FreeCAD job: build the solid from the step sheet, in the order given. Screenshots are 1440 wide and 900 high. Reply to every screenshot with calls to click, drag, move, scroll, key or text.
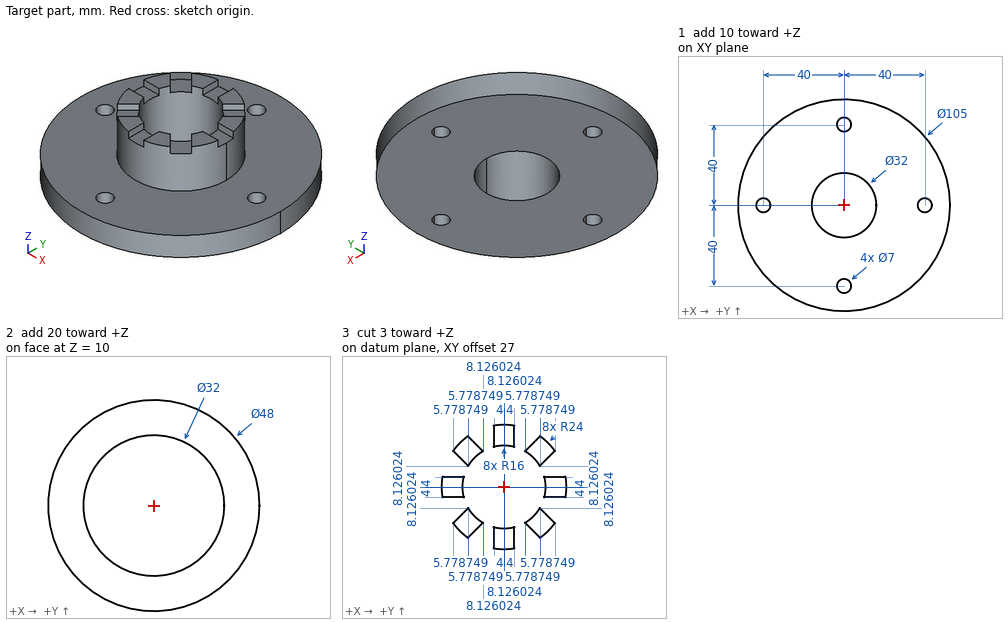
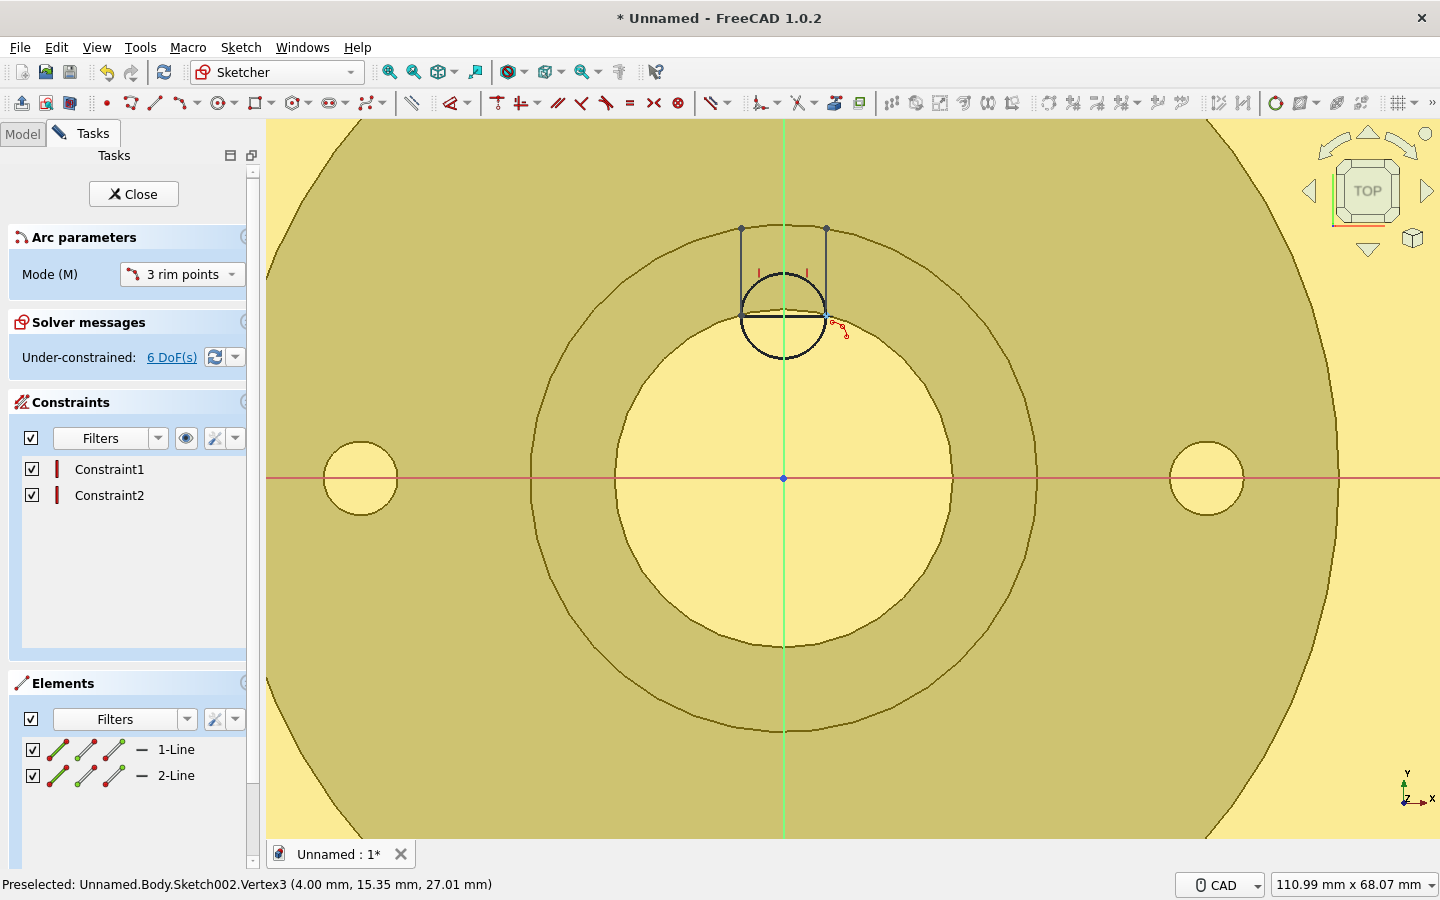
scroll(792, 309, up, 6)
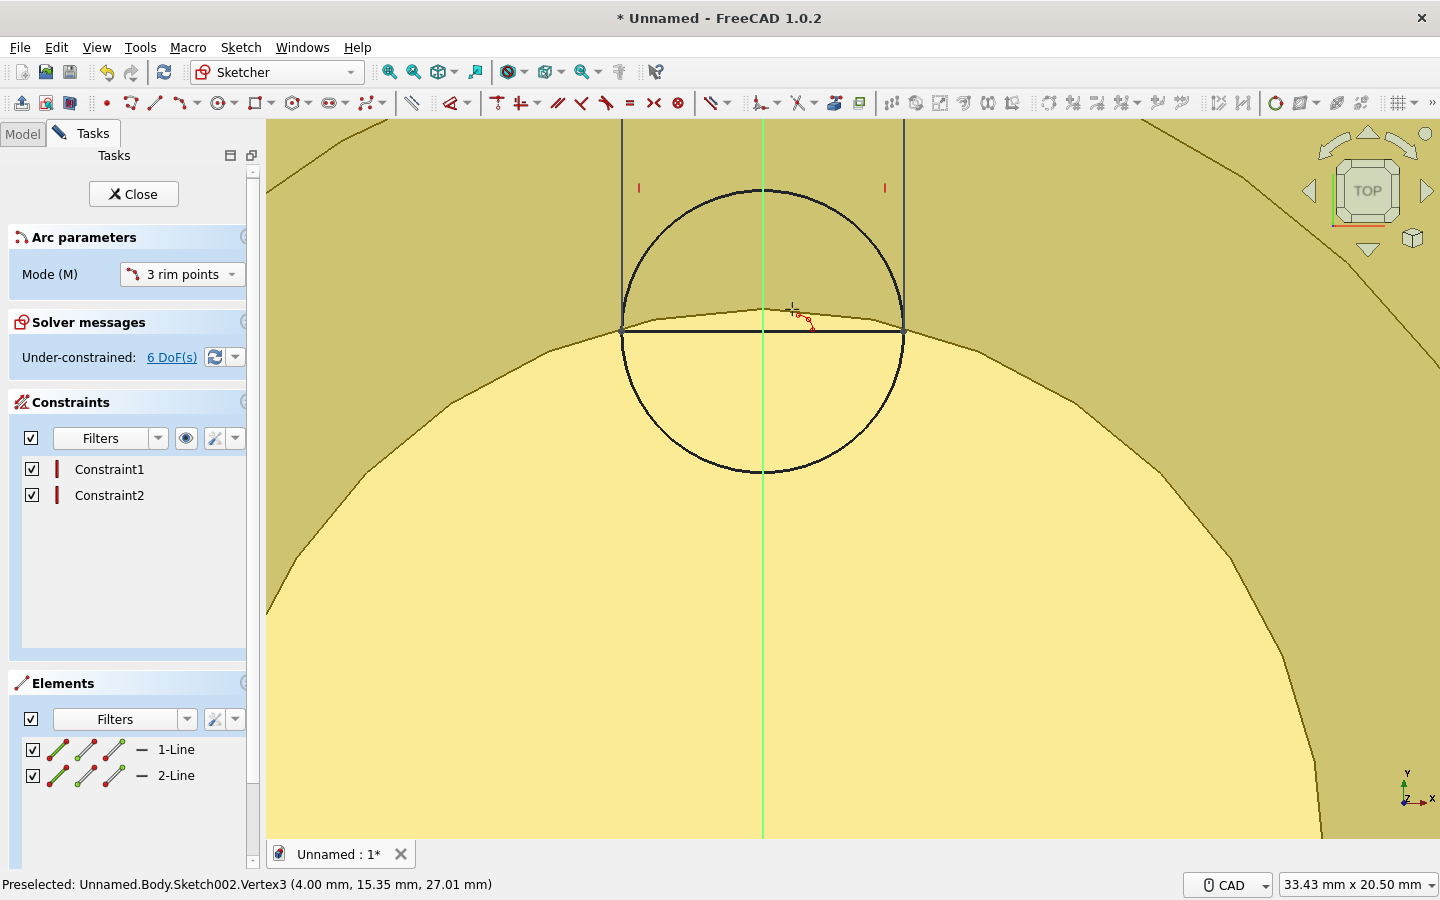
click(792, 310)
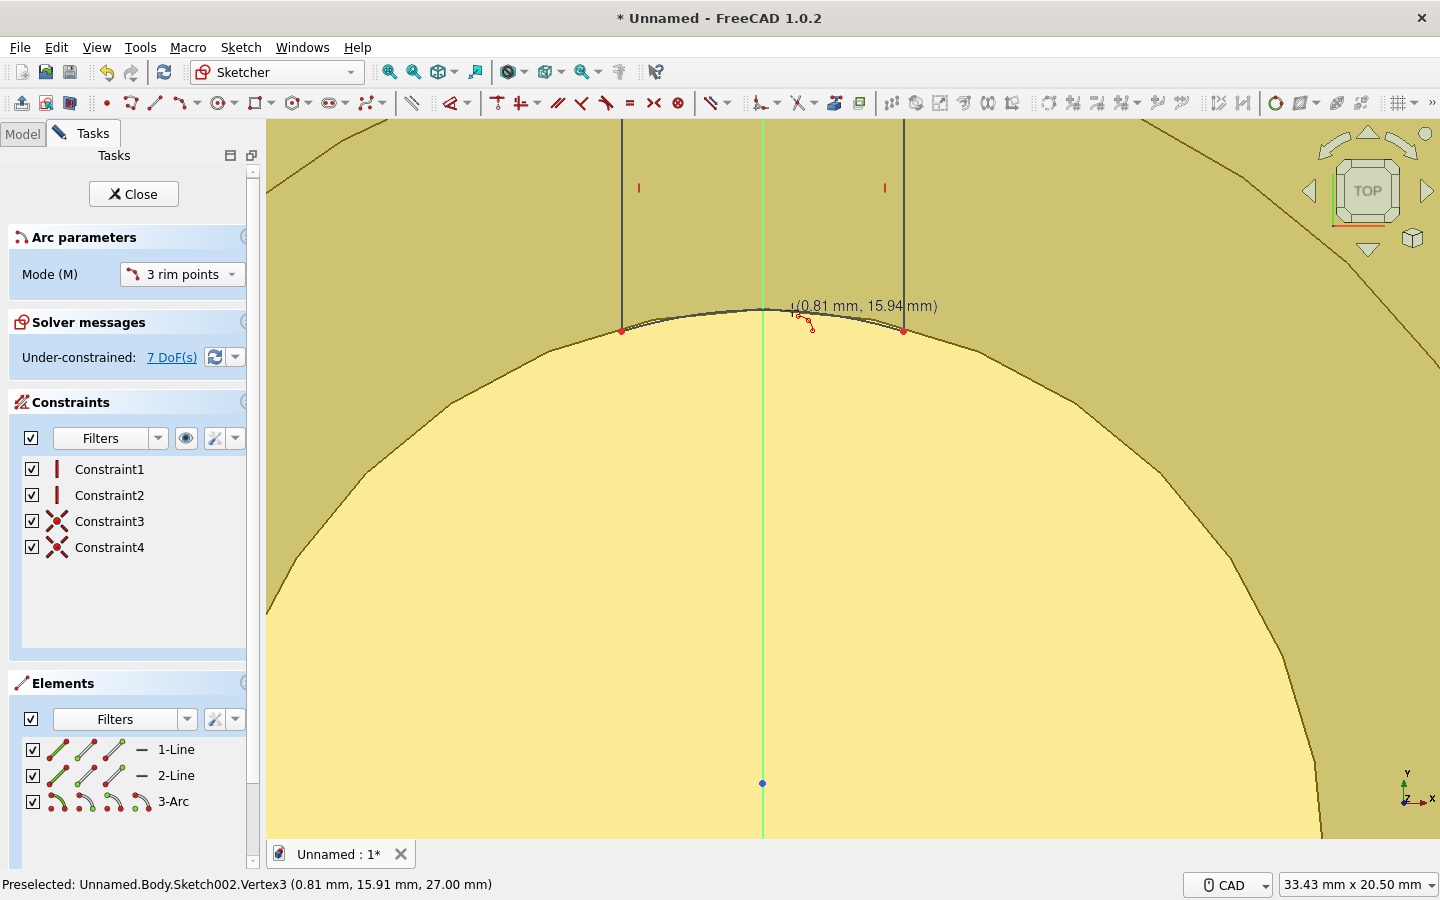
scroll(794, 310, down, 6)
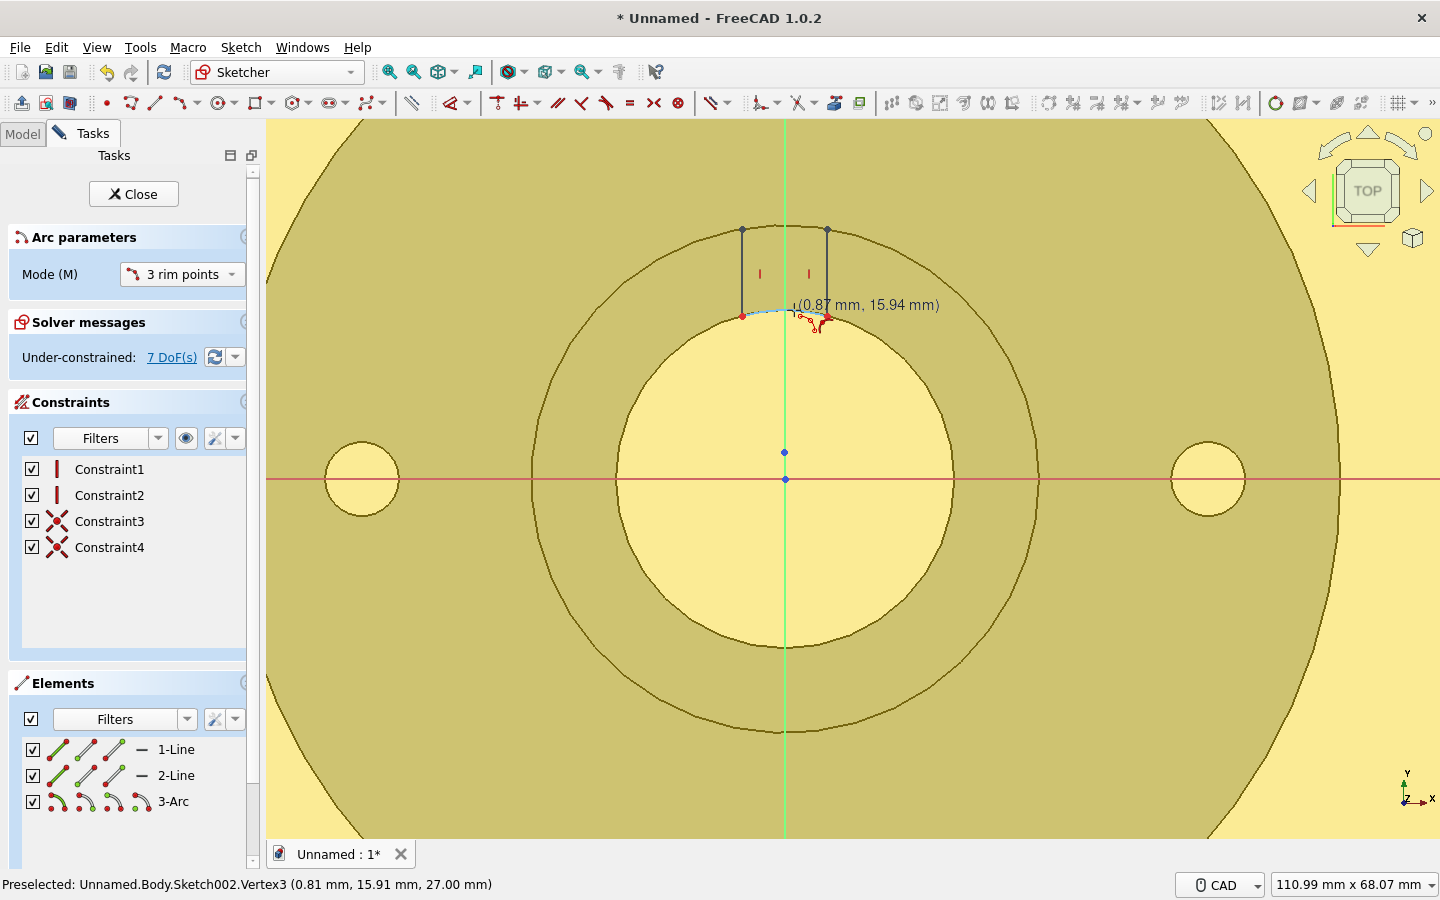
click(827, 230)
click(742, 230)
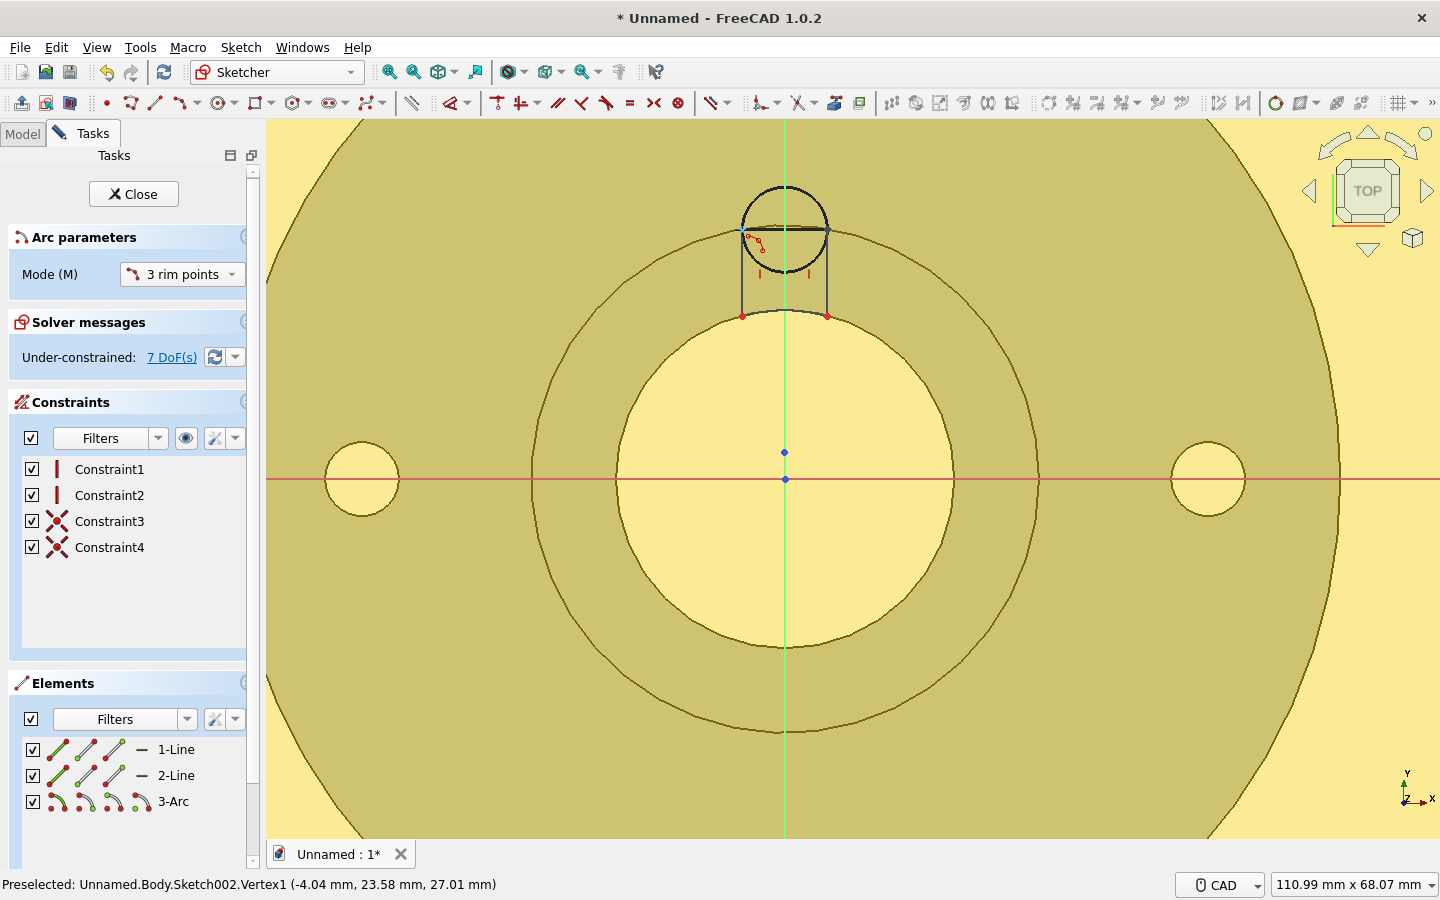
scroll(794, 225, up, 8)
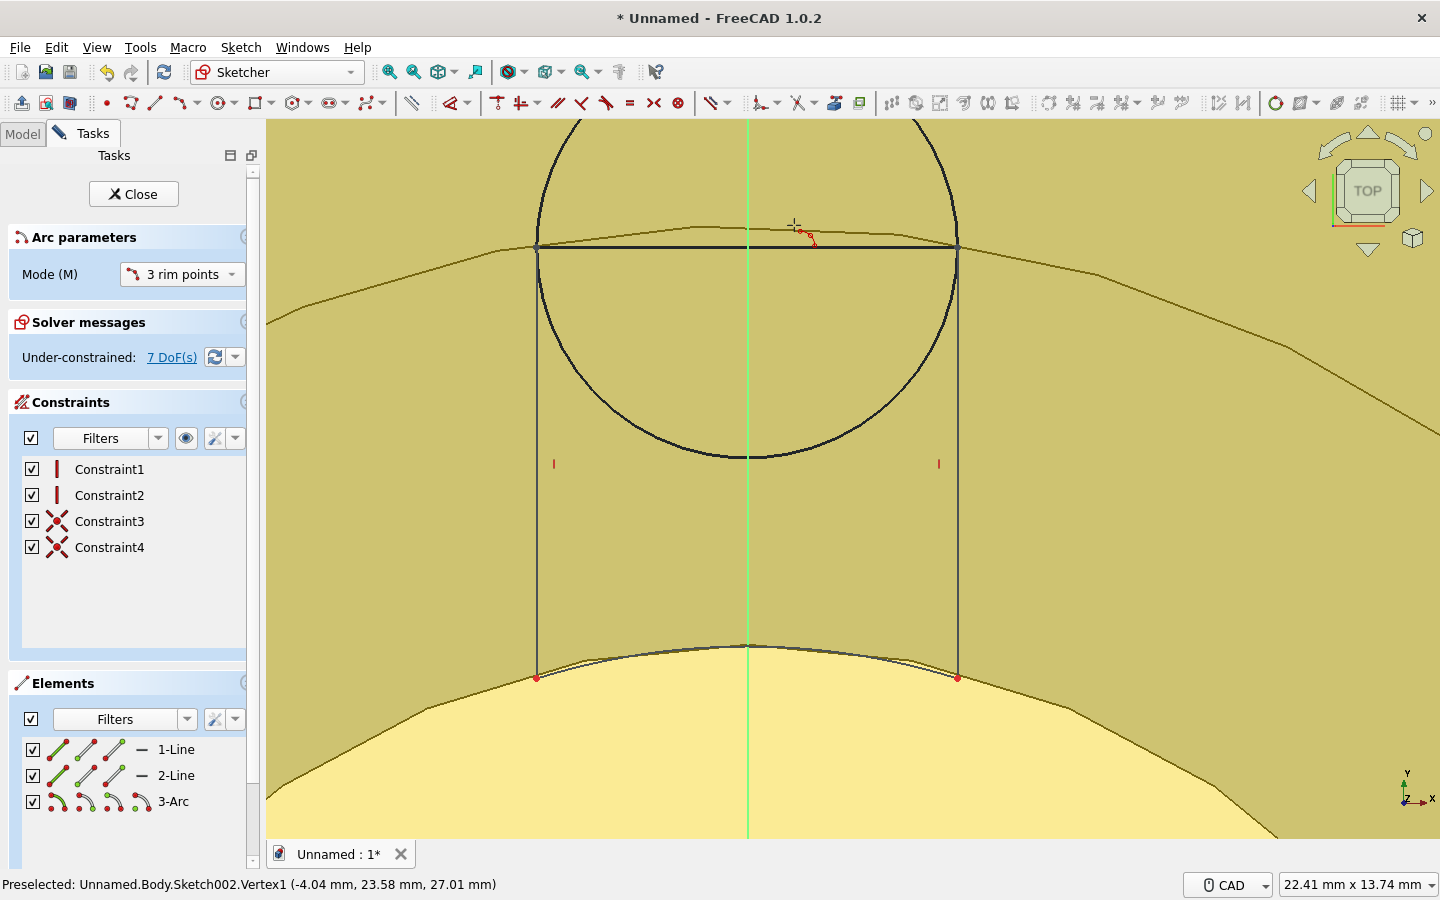
click(790, 226)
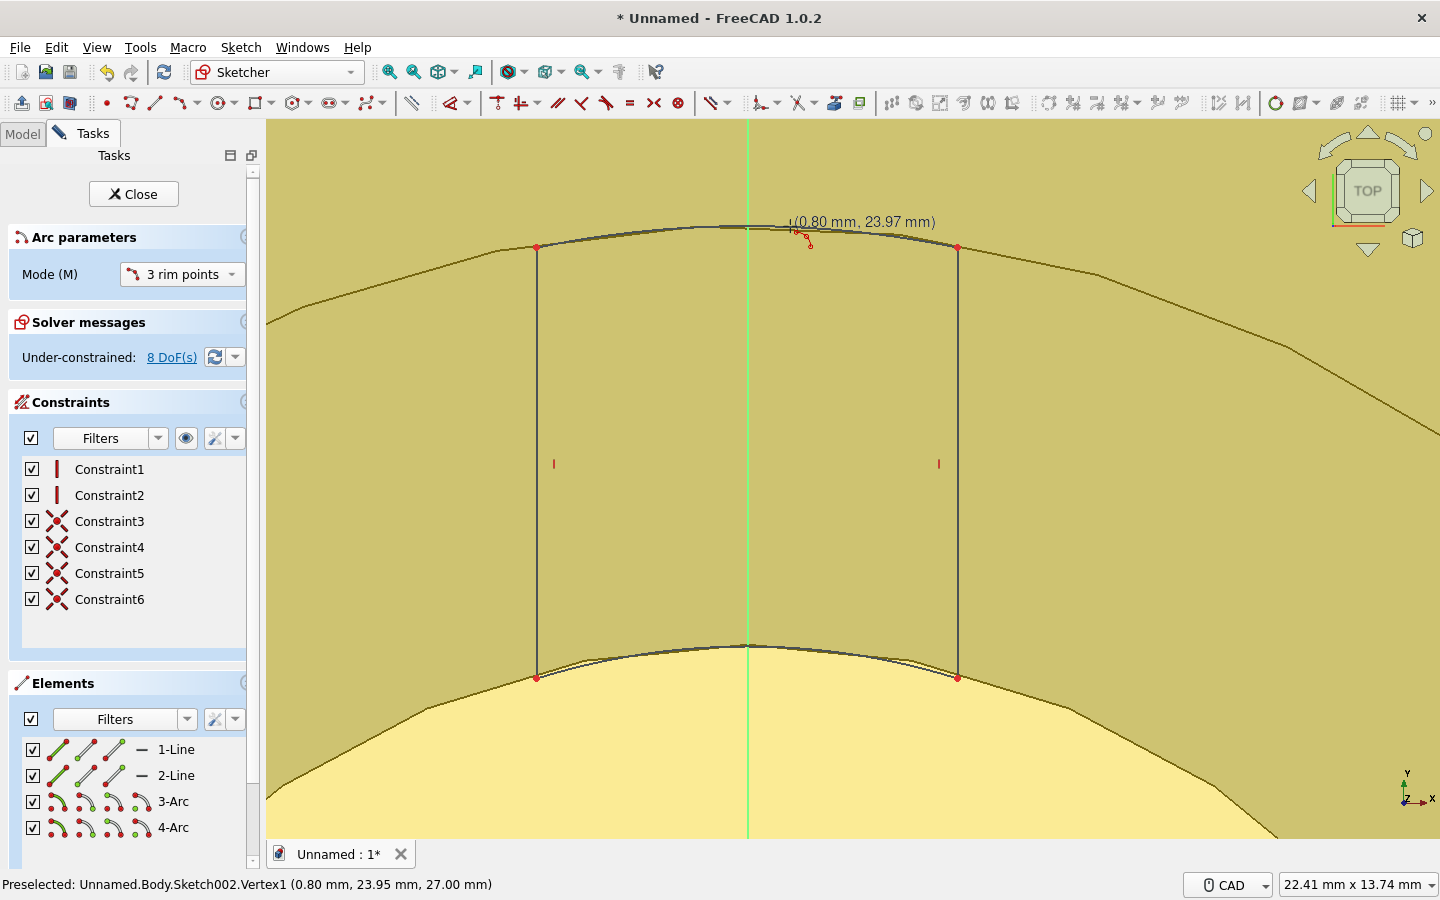
click(156, 104)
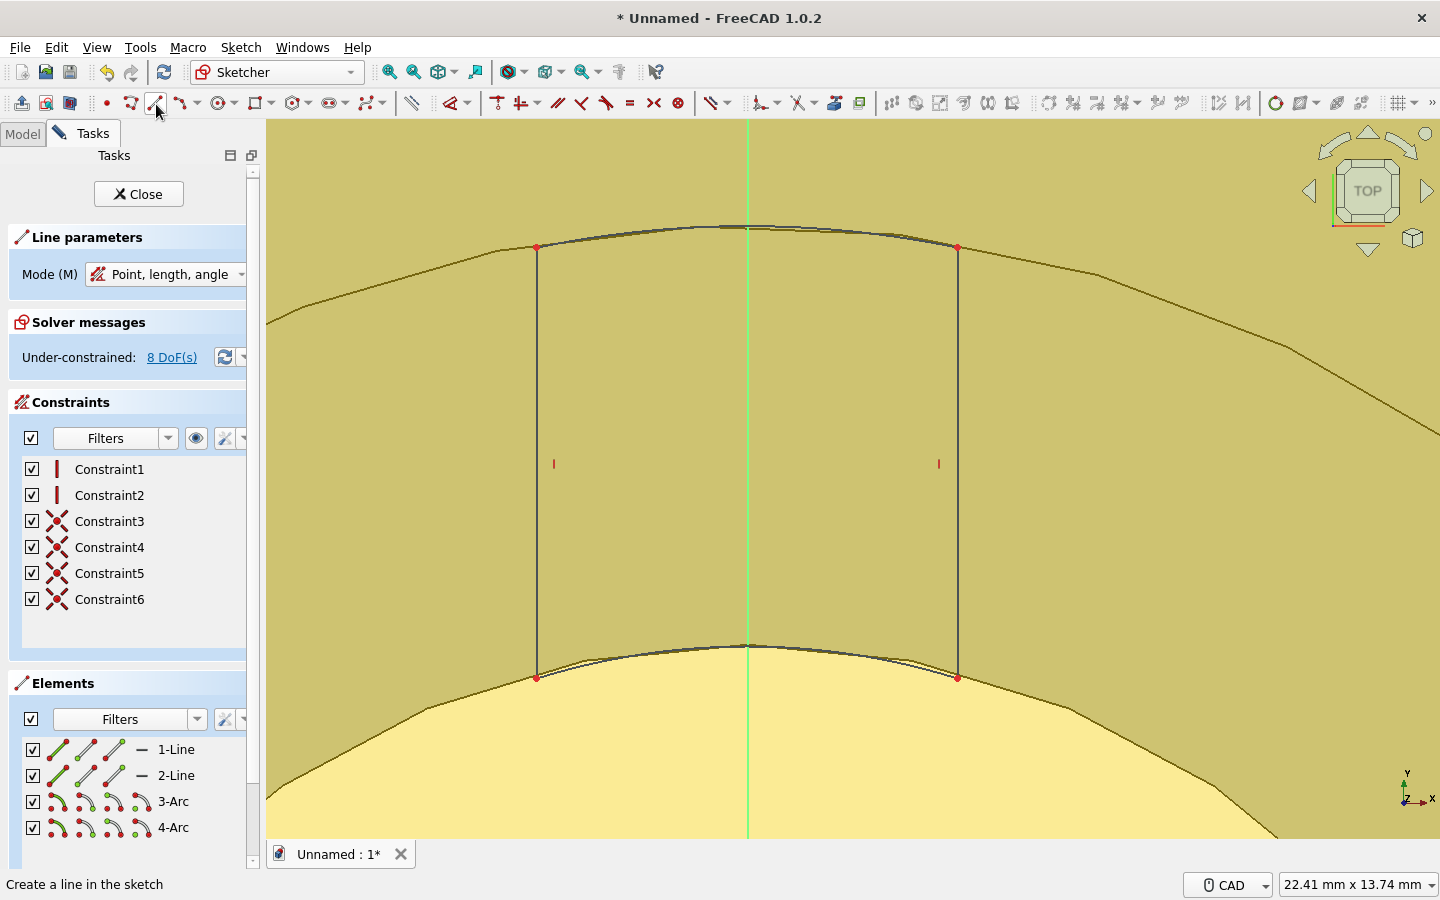
scroll(794, 225, down, 8)